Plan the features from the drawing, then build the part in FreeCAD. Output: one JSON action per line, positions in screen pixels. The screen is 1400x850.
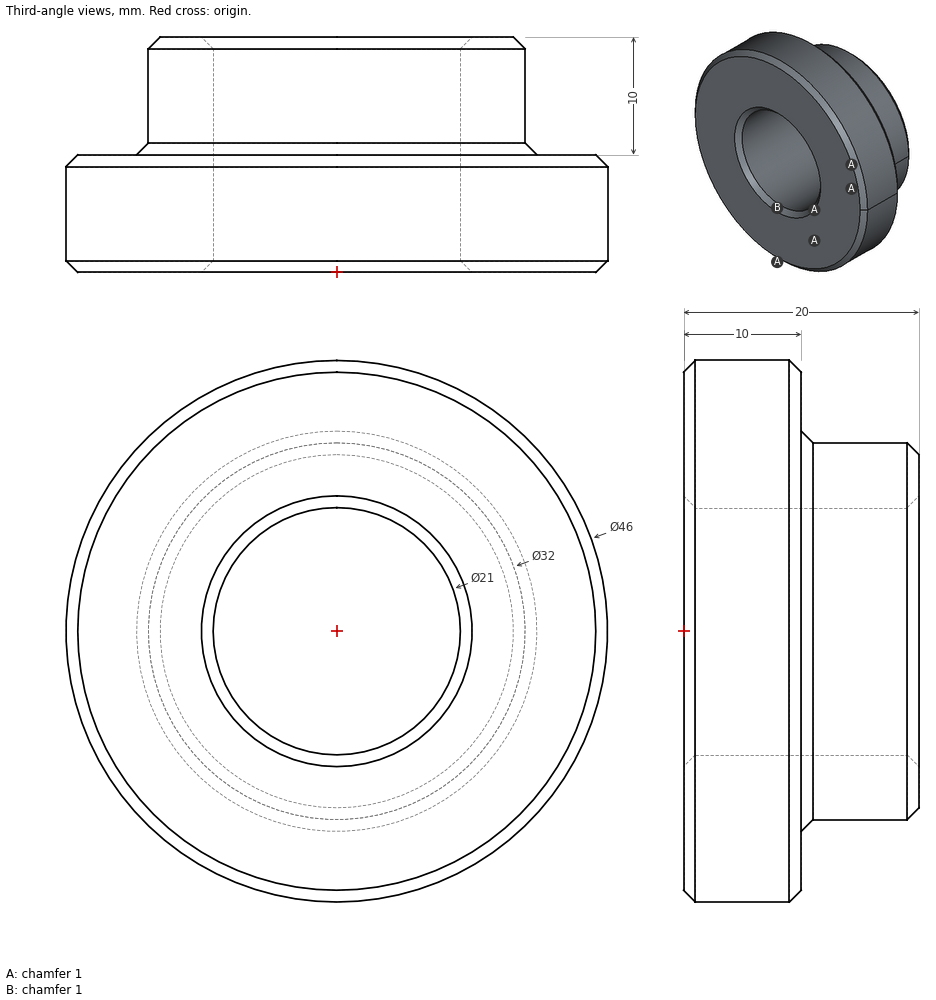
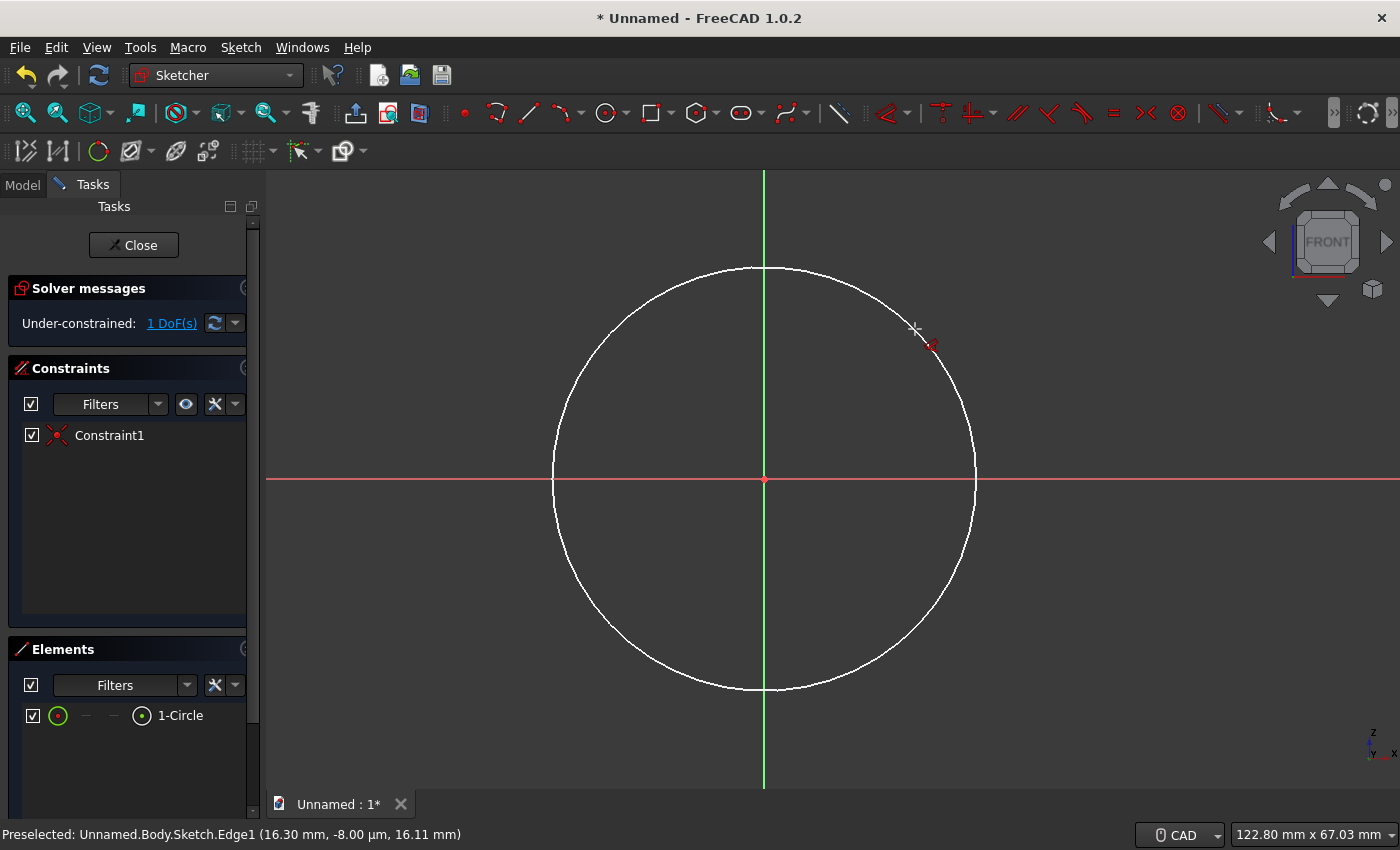
{"action": "left_click", "coordinate": [914, 329]}
{"action": "left_click", "coordinate": [937, 306]}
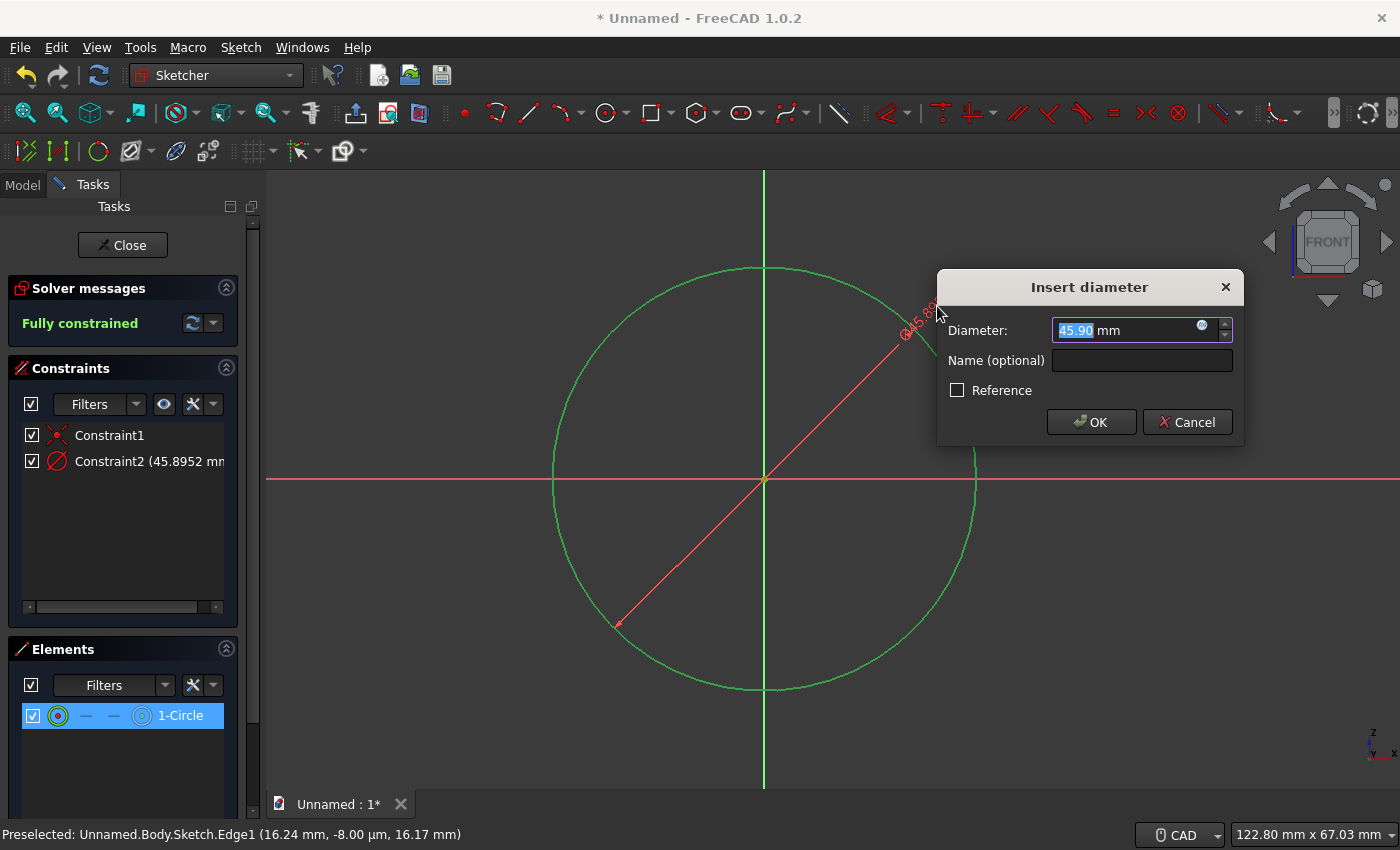
{"action": "type", "text": "46"}
{"action": "key", "text": "Return"}
{"action": "key", "text": "Escape"}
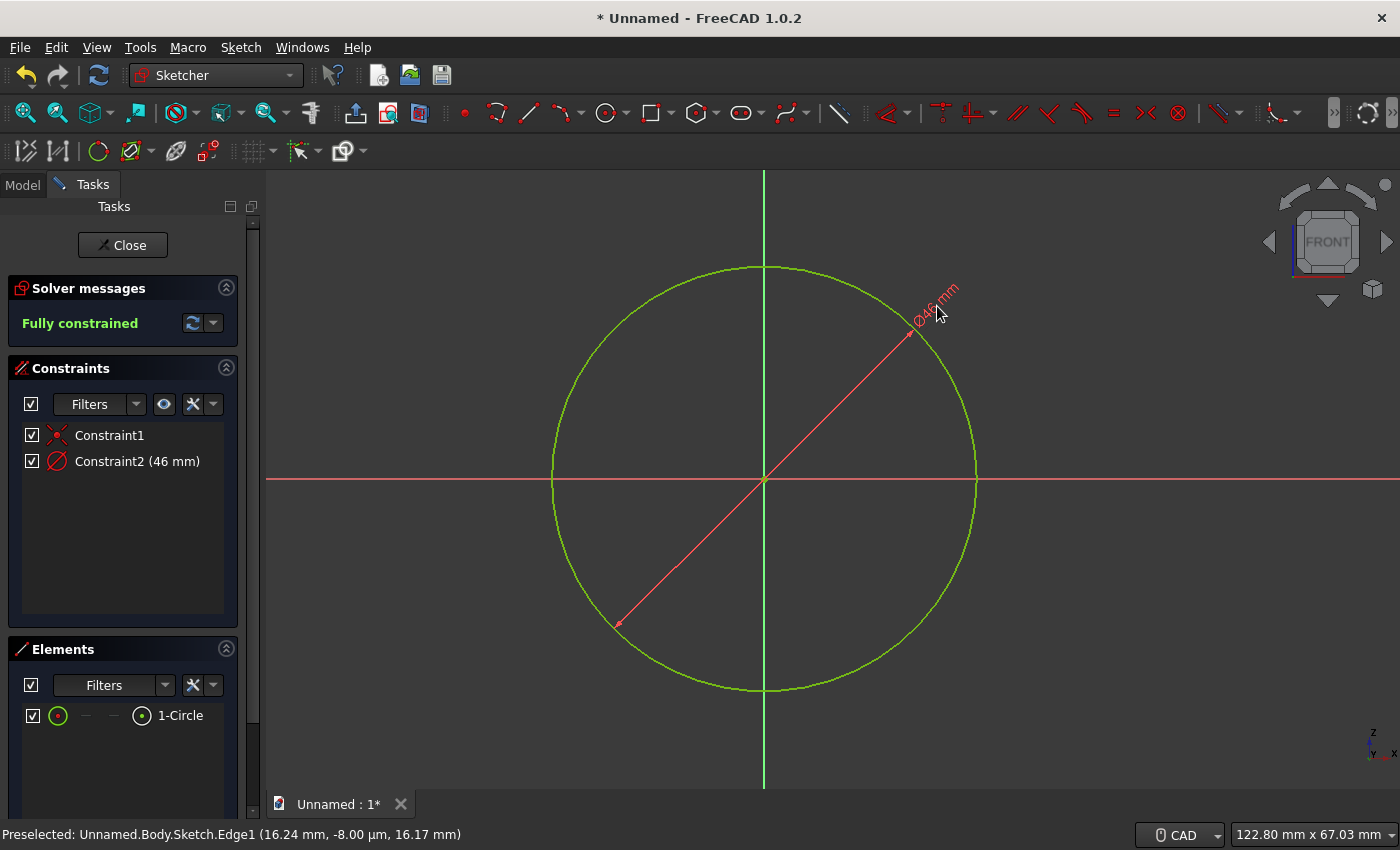
{"action": "left_click", "coordinate": [123, 245]}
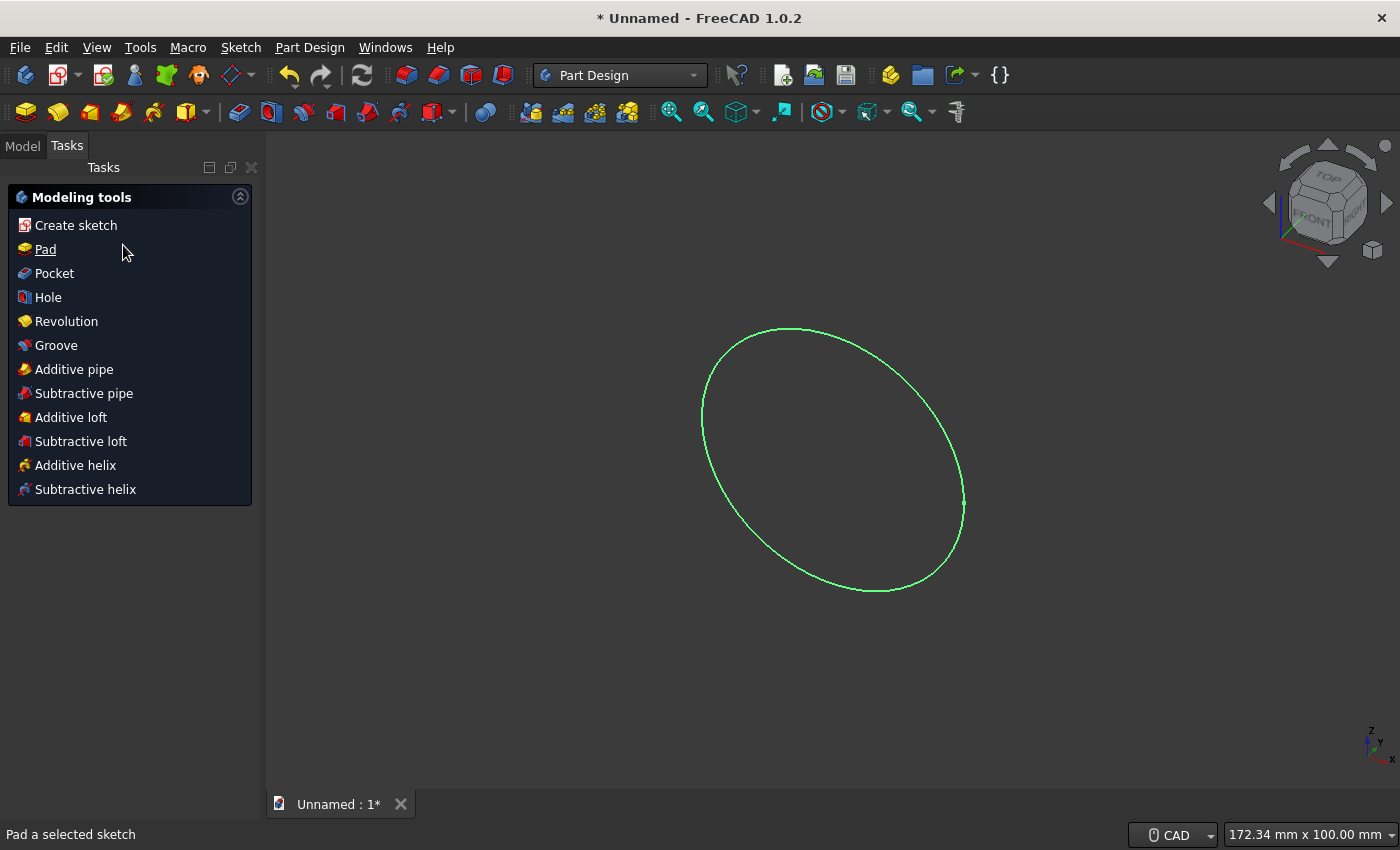
{"action": "left_click", "coordinate": [26, 112]}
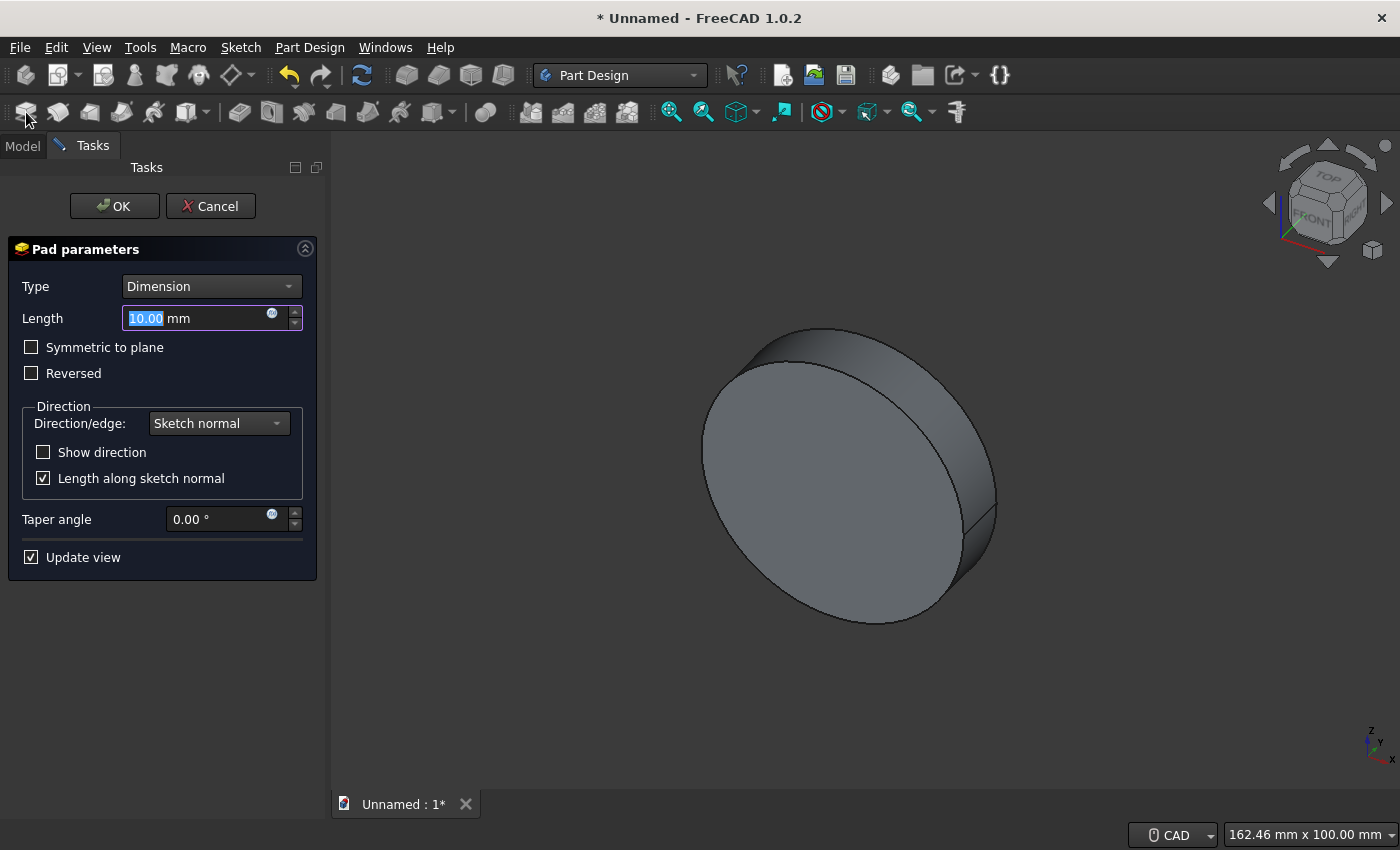
{"action": "type", "text": "10"}
{"action": "key", "text": "Tab"}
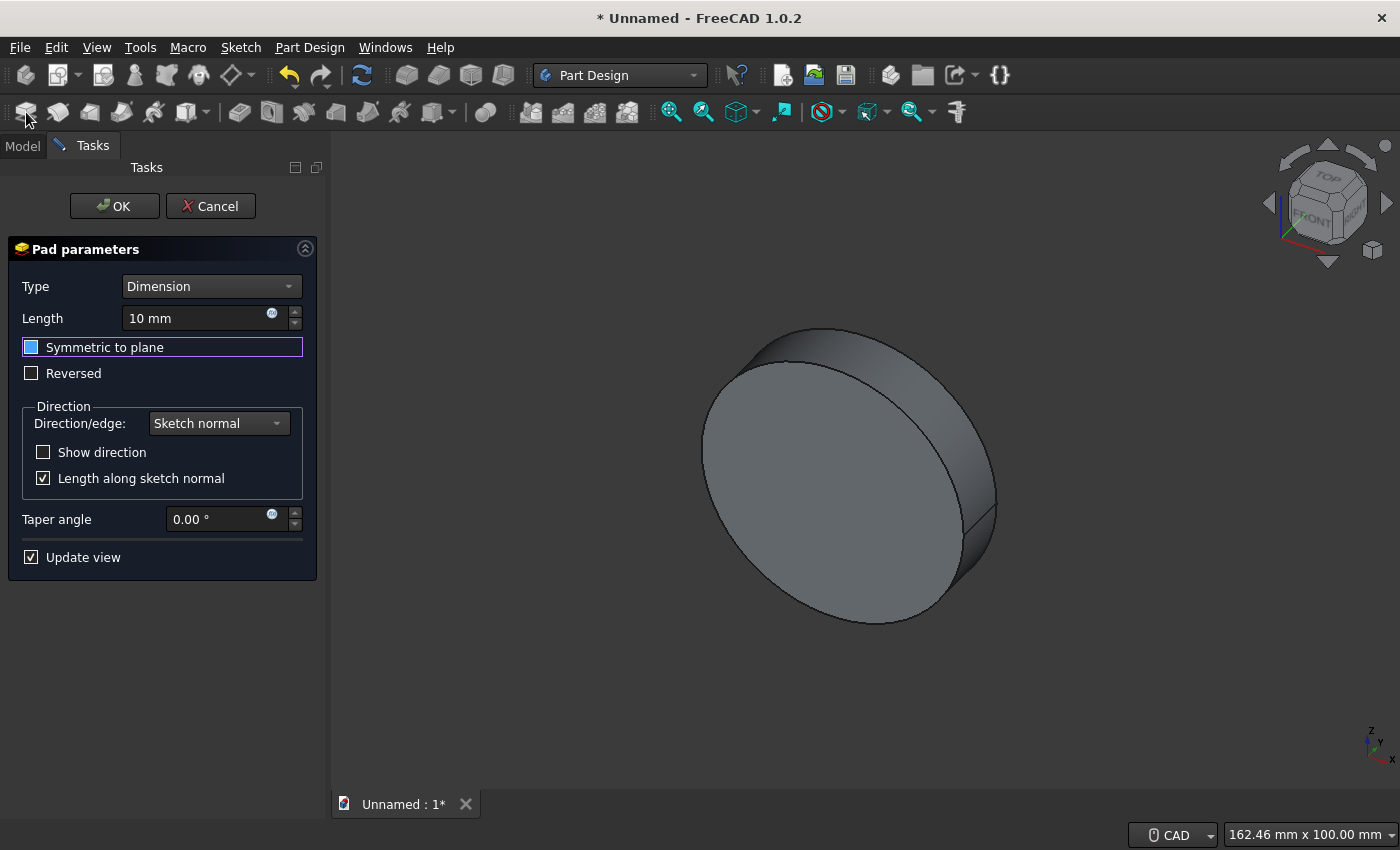
{"action": "left_click", "coordinate": [30, 373]}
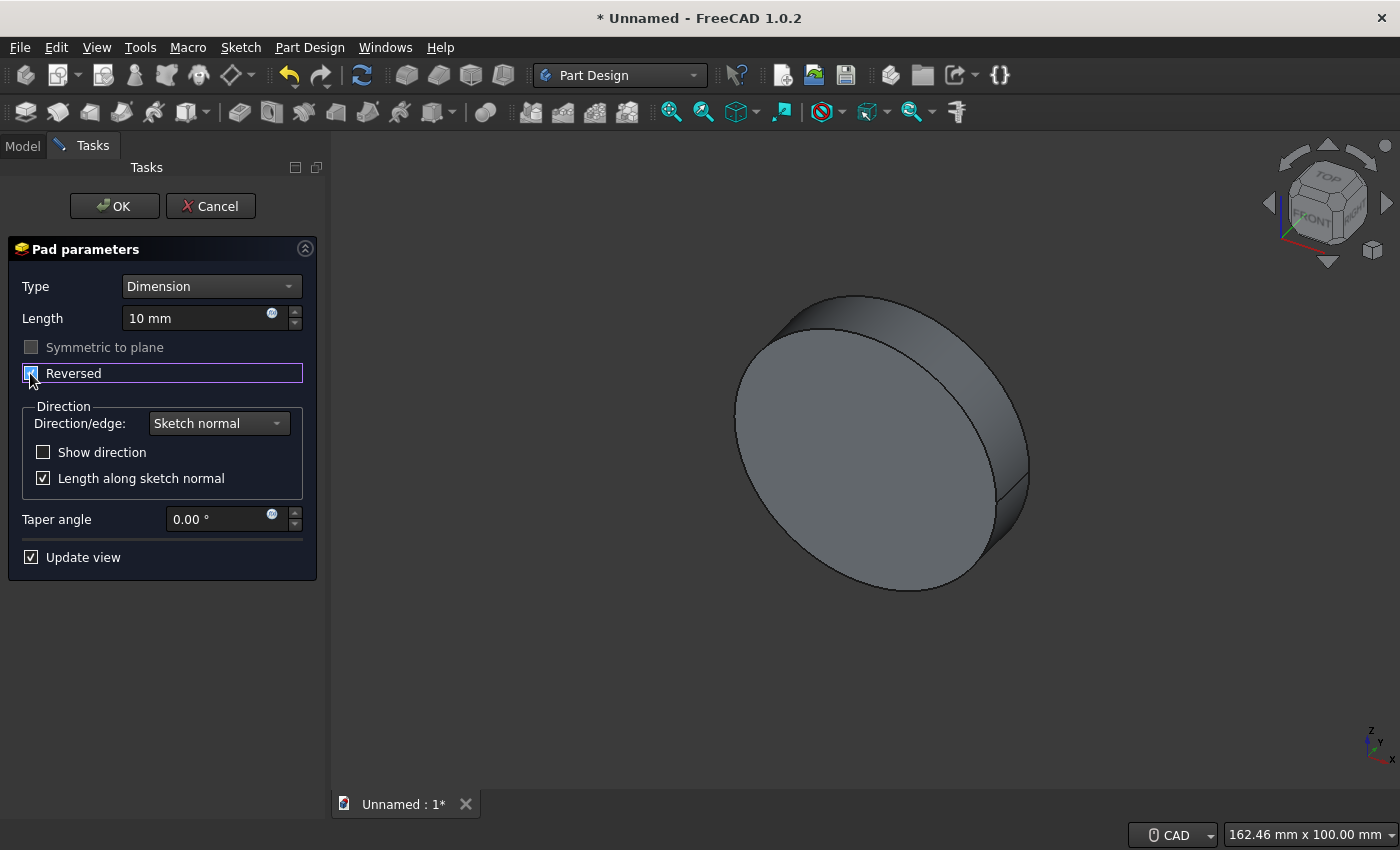
{"action": "left_click", "coordinate": [115, 206]}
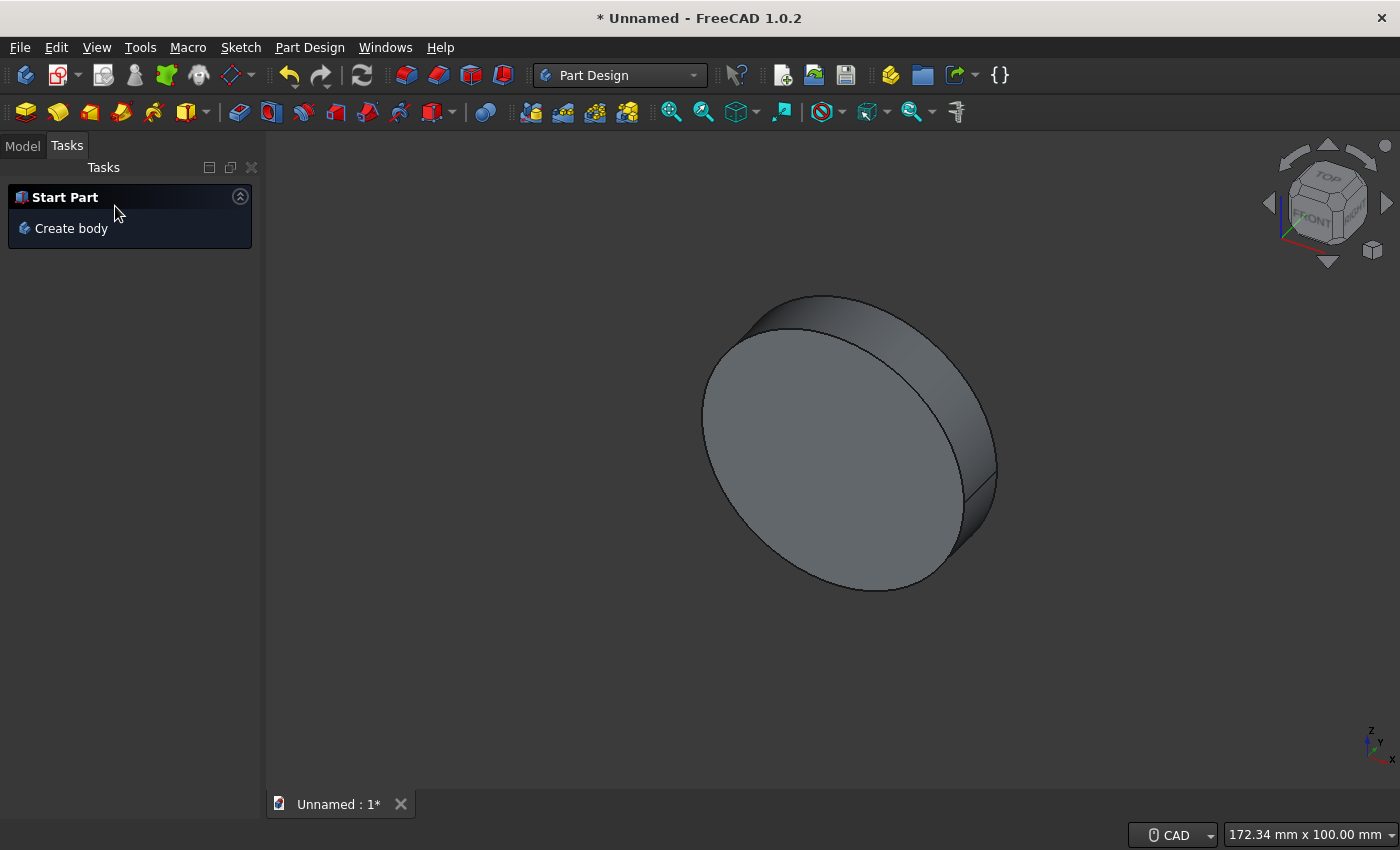
{"action": "key", "text": "4"}